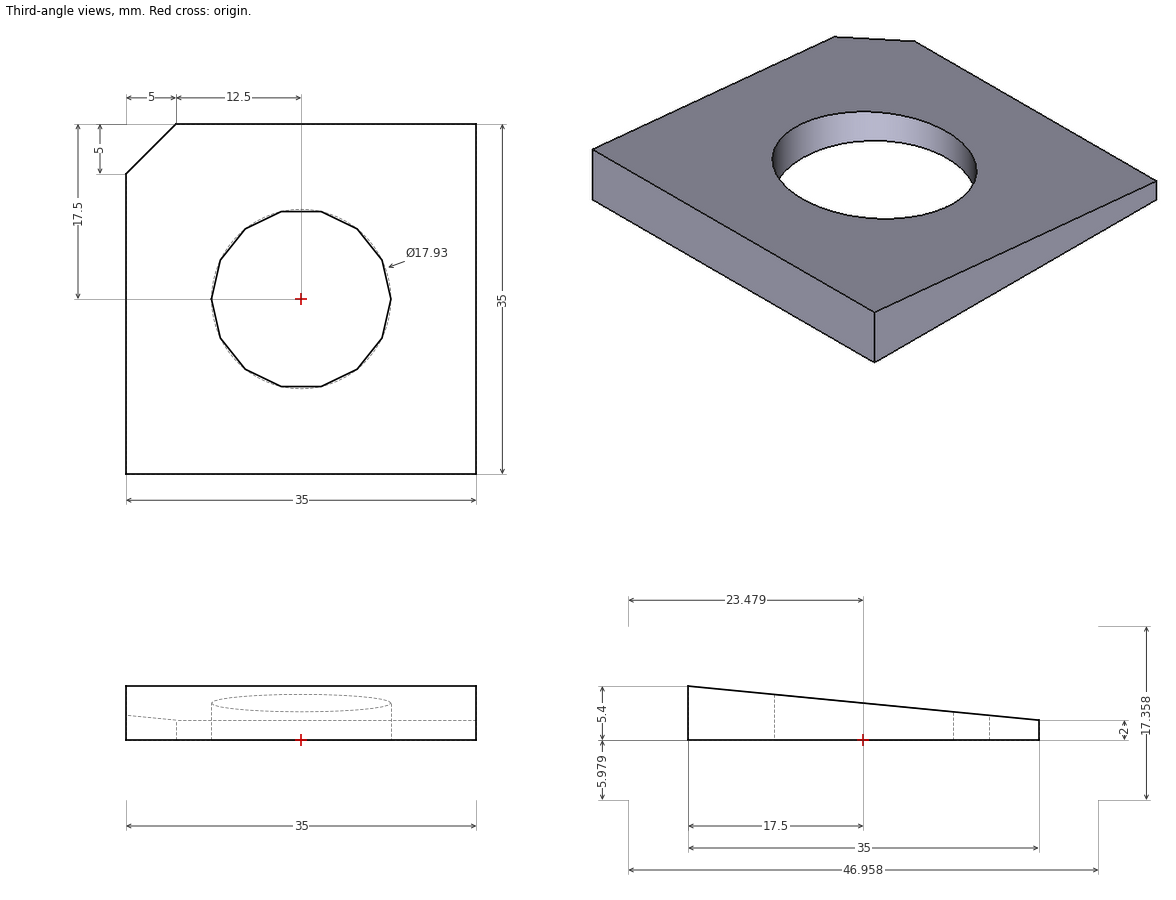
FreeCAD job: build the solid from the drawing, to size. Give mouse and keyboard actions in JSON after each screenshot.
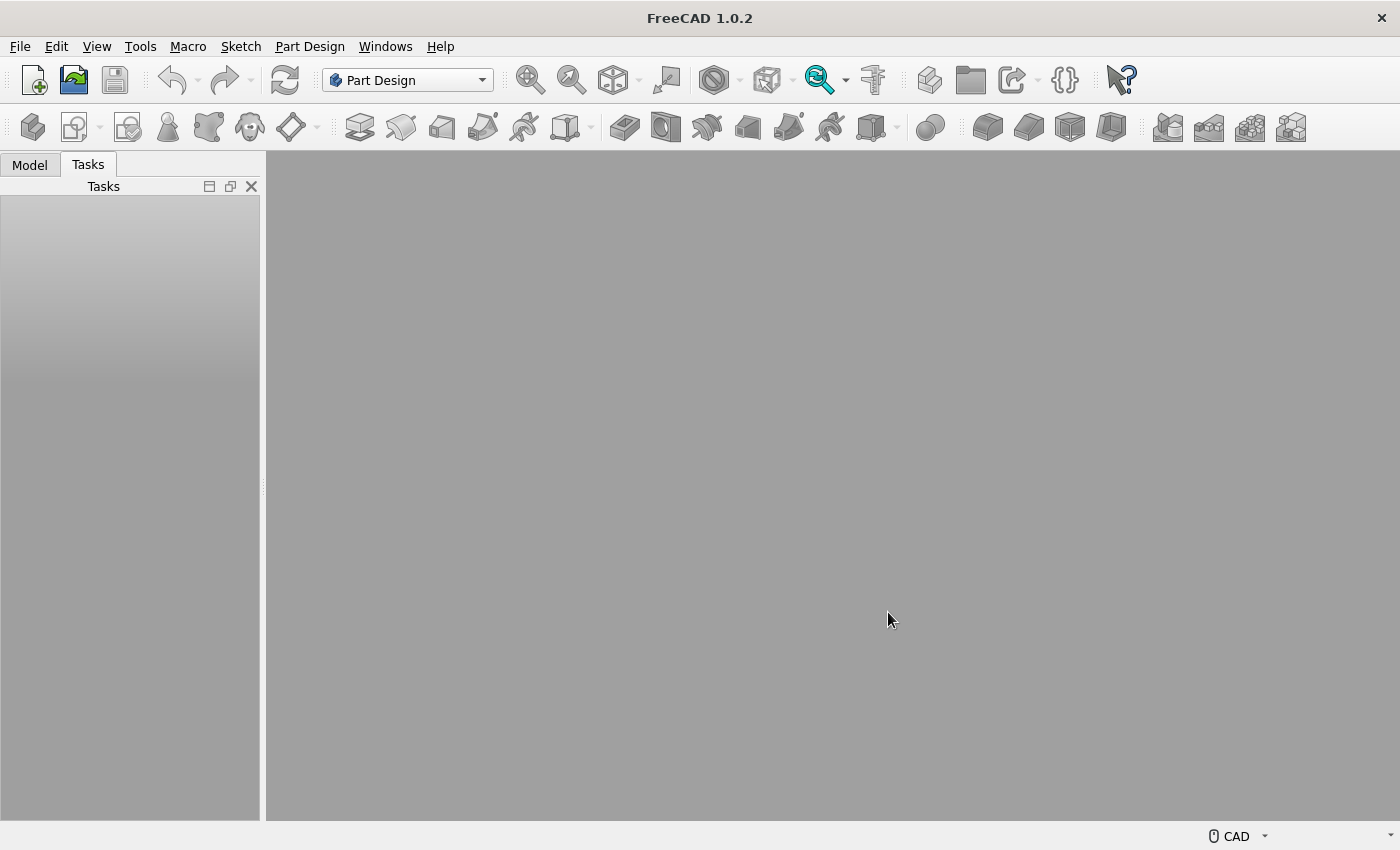
{"action": "key", "text": "ctrl+n"}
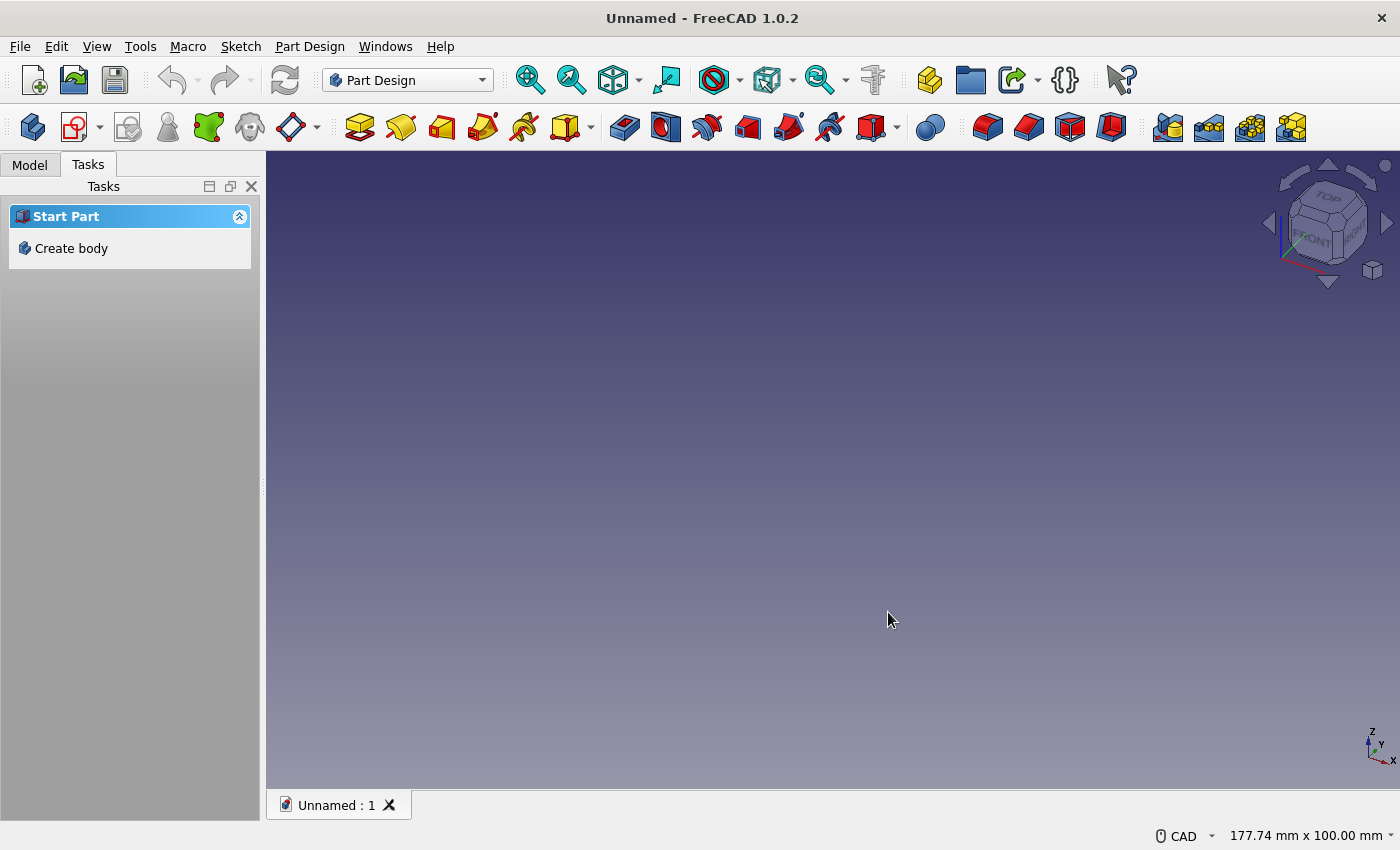
{"action": "left_click", "coordinate": [74, 128]}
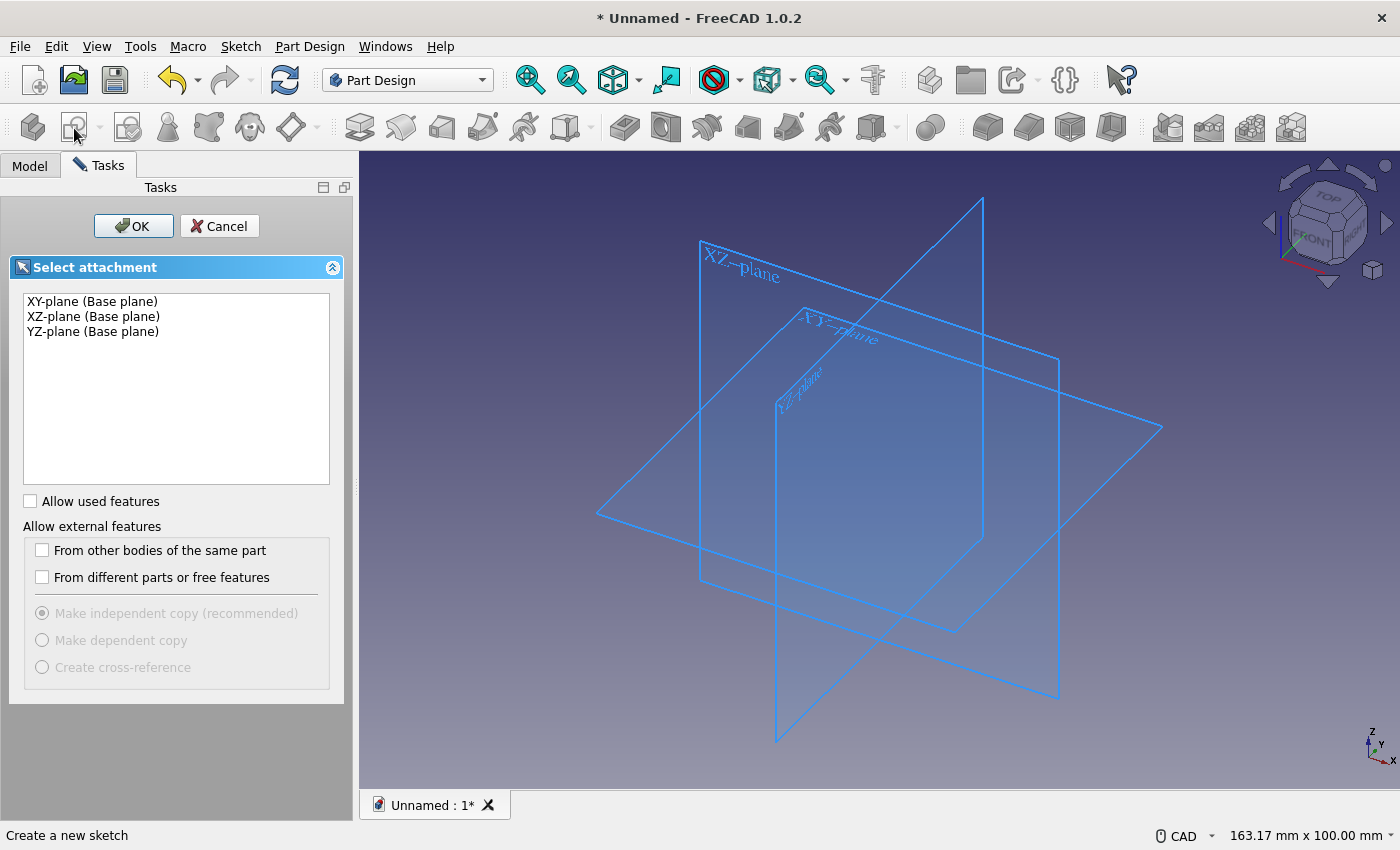
{"action": "left_click", "coordinate": [84, 302]}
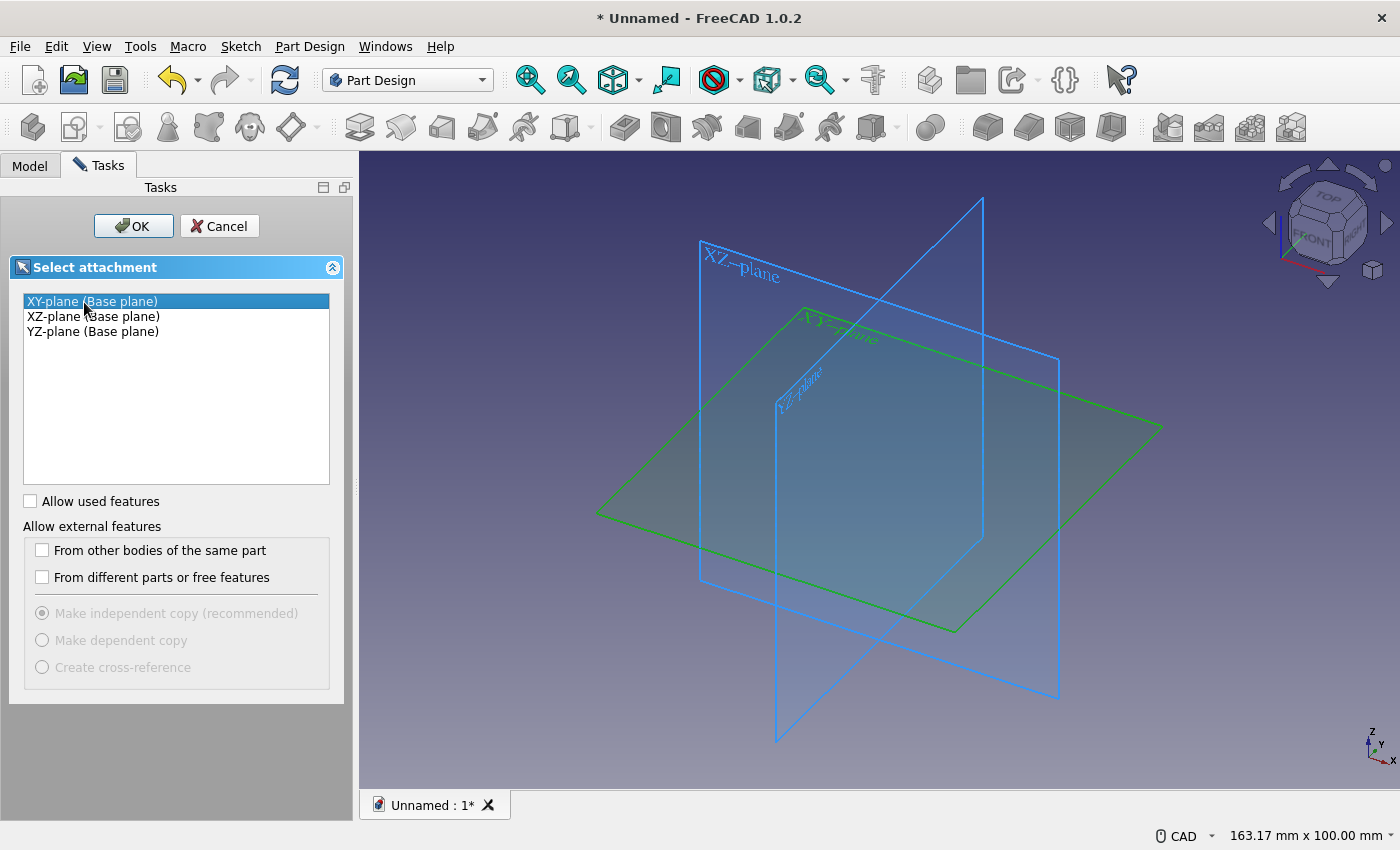
{"action": "left_click", "coordinate": [134, 226]}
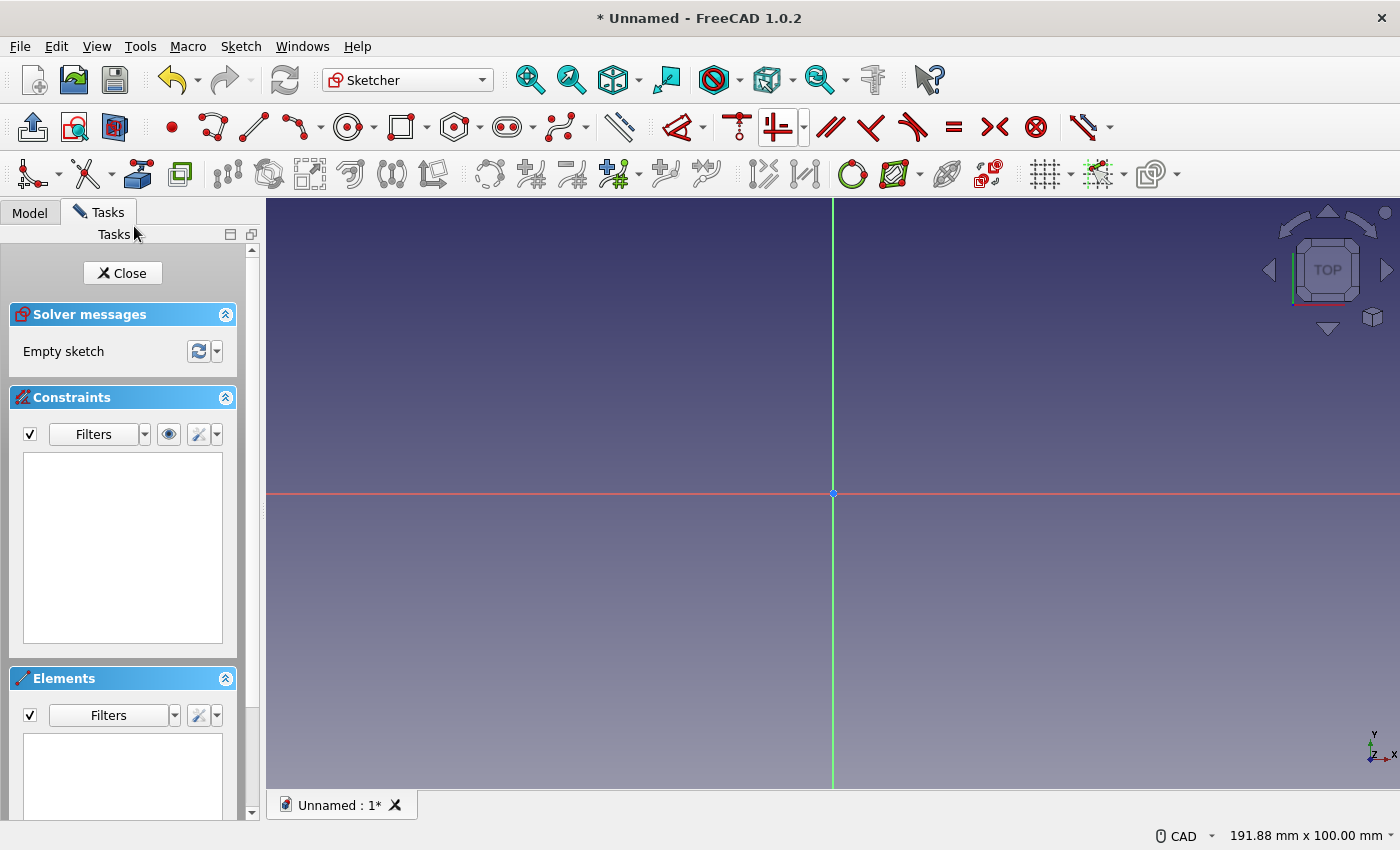
{"action": "scroll", "coordinate": [916, 494], "scroll_direction": "up", "scroll_amount": 3}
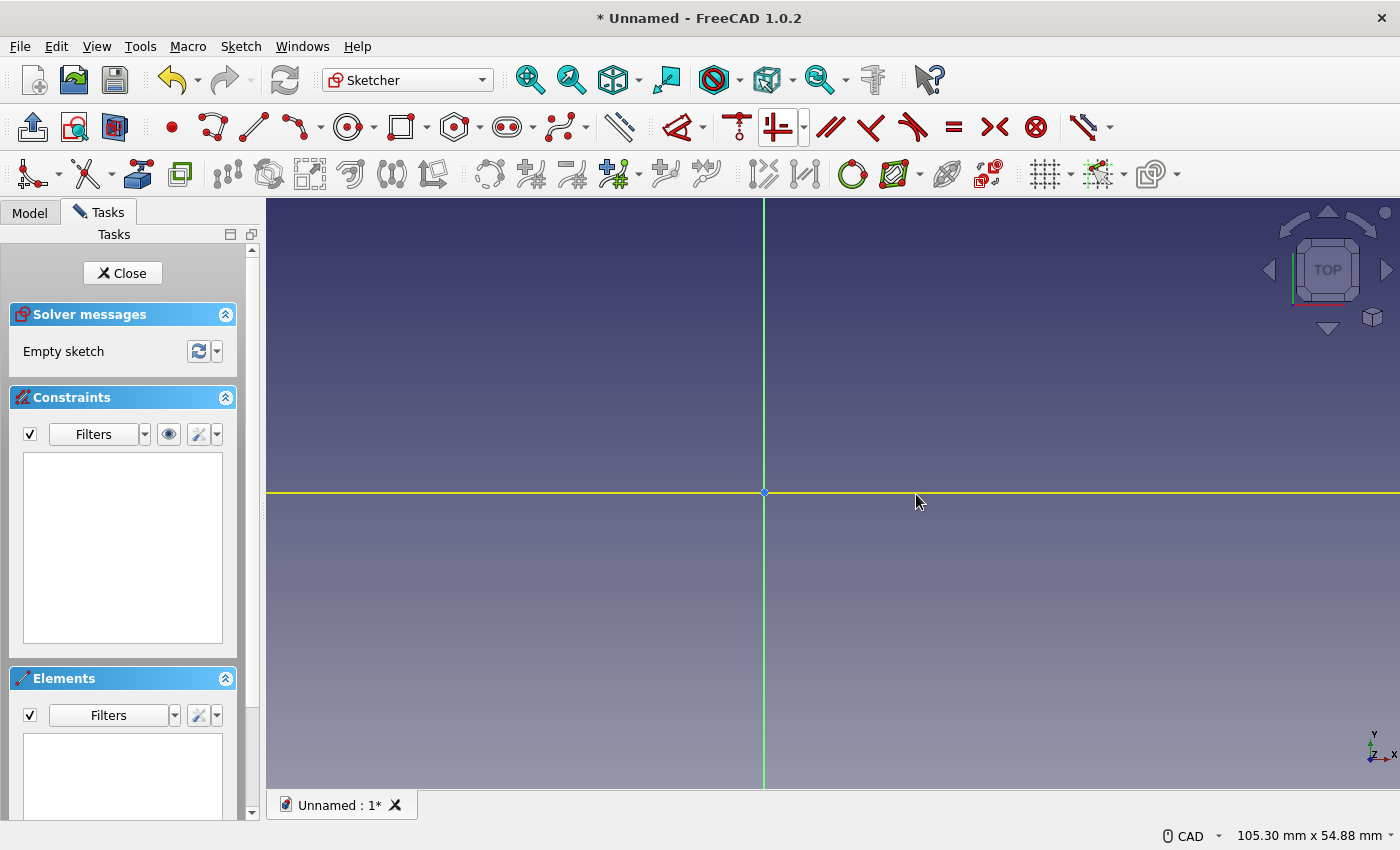
{"action": "left_click", "coordinate": [426, 128]}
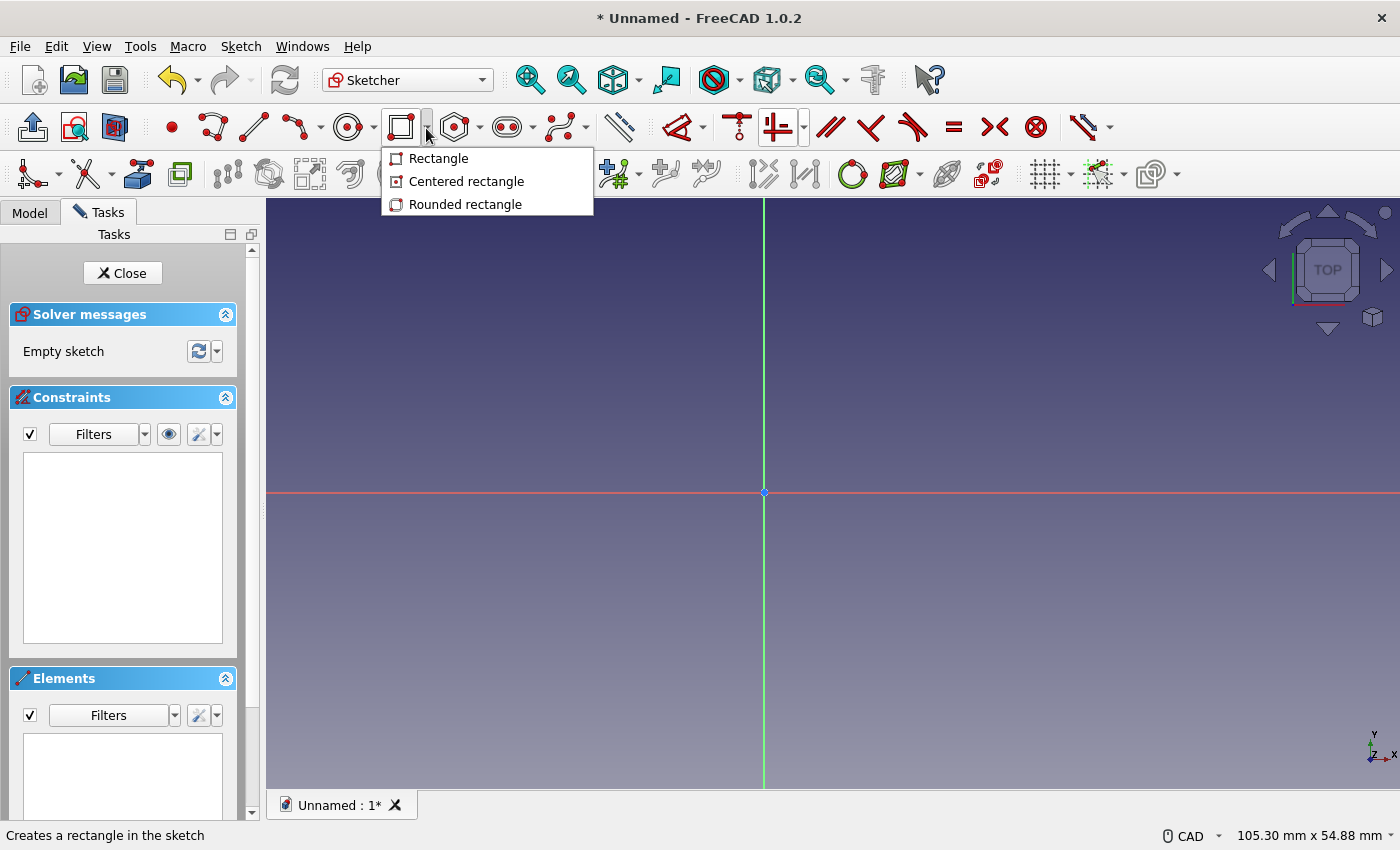
{"action": "left_click", "coordinate": [488, 182]}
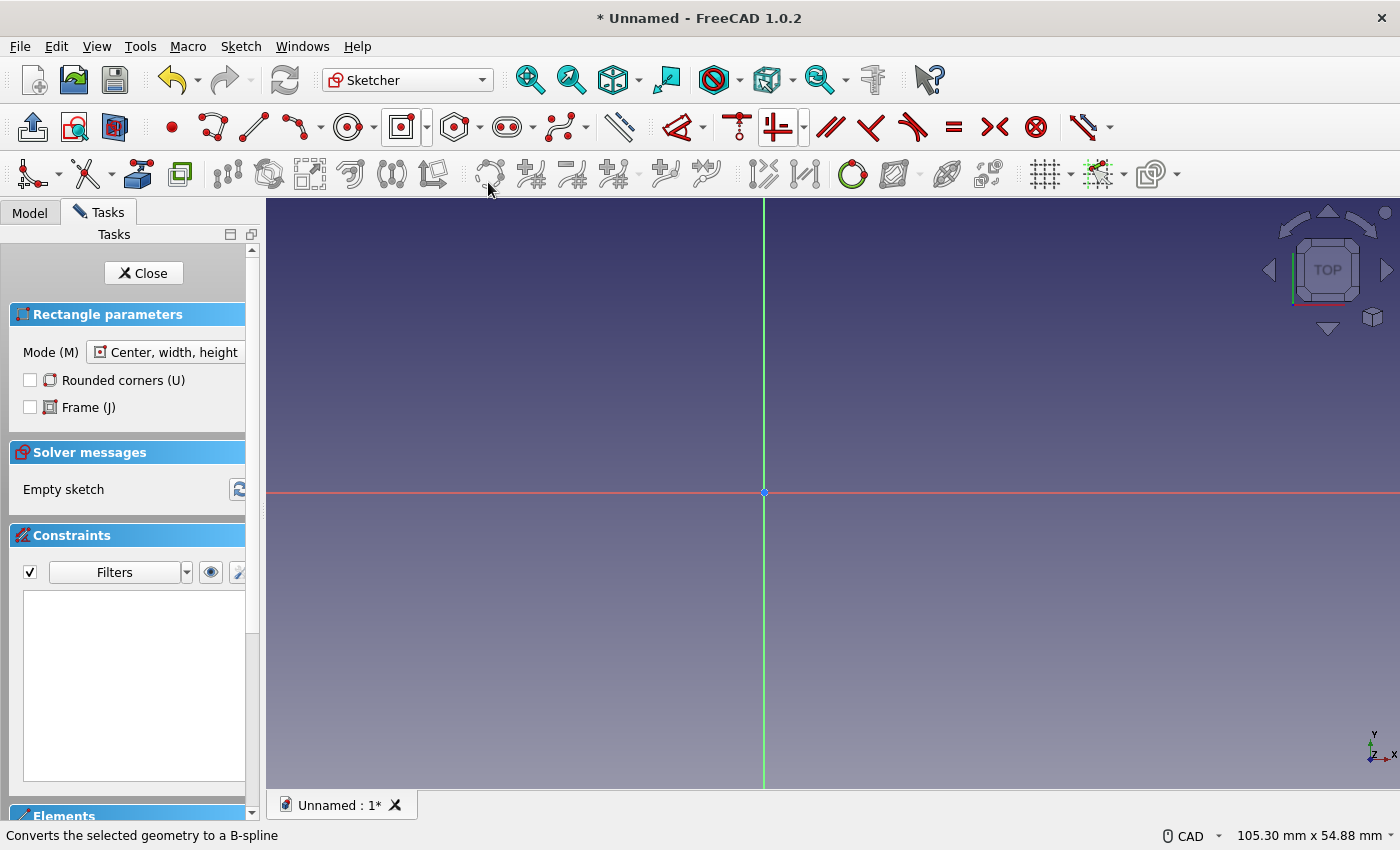
{"action": "left_click", "coordinate": [764, 493]}
{"action": "mouse_move", "coordinate": [953, 304]}